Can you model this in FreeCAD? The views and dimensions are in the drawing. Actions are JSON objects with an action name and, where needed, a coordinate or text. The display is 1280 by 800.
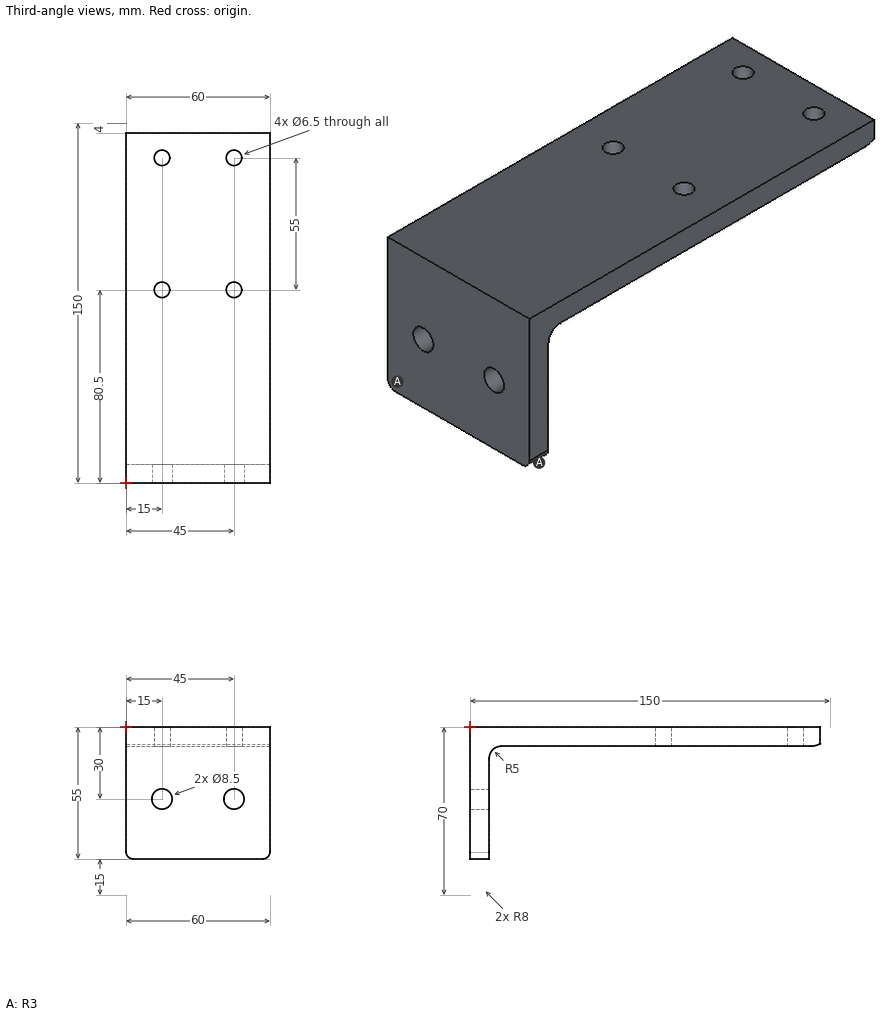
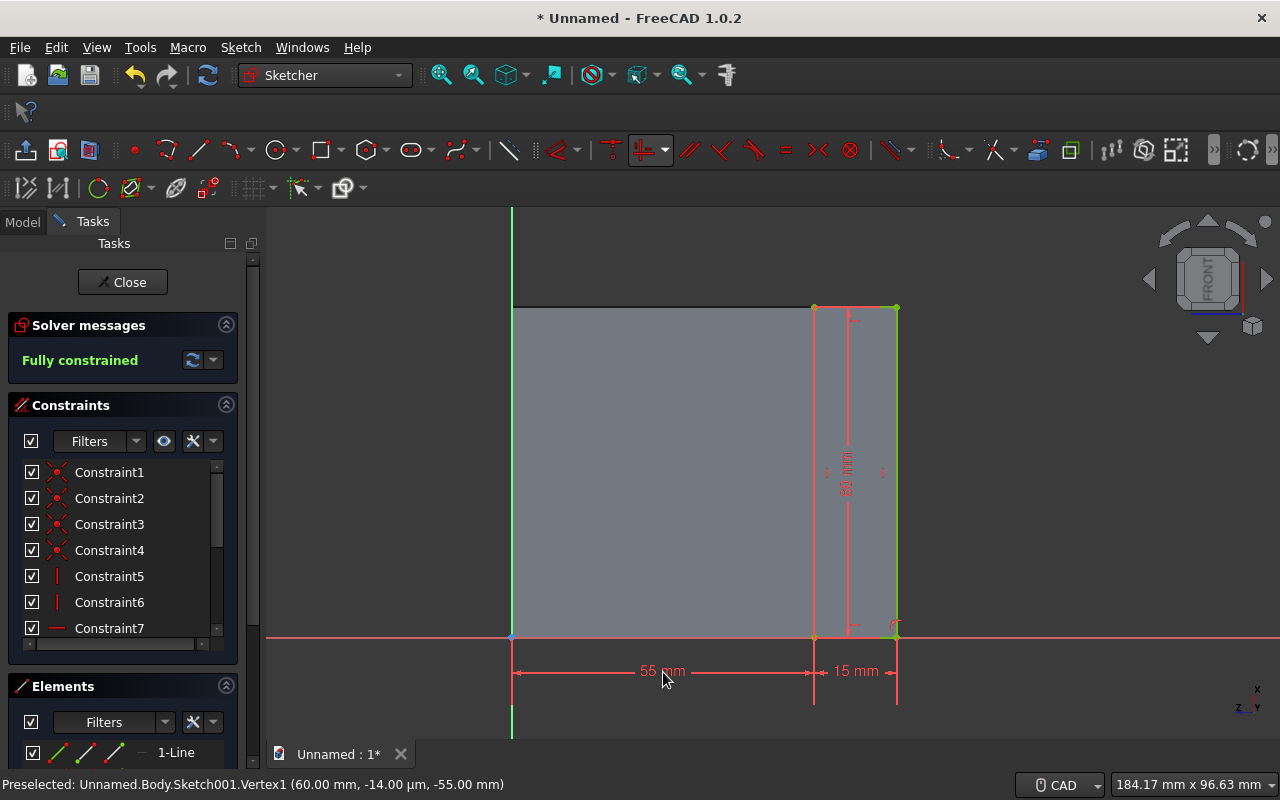
{"action": "left_click", "coordinate": [123, 282]}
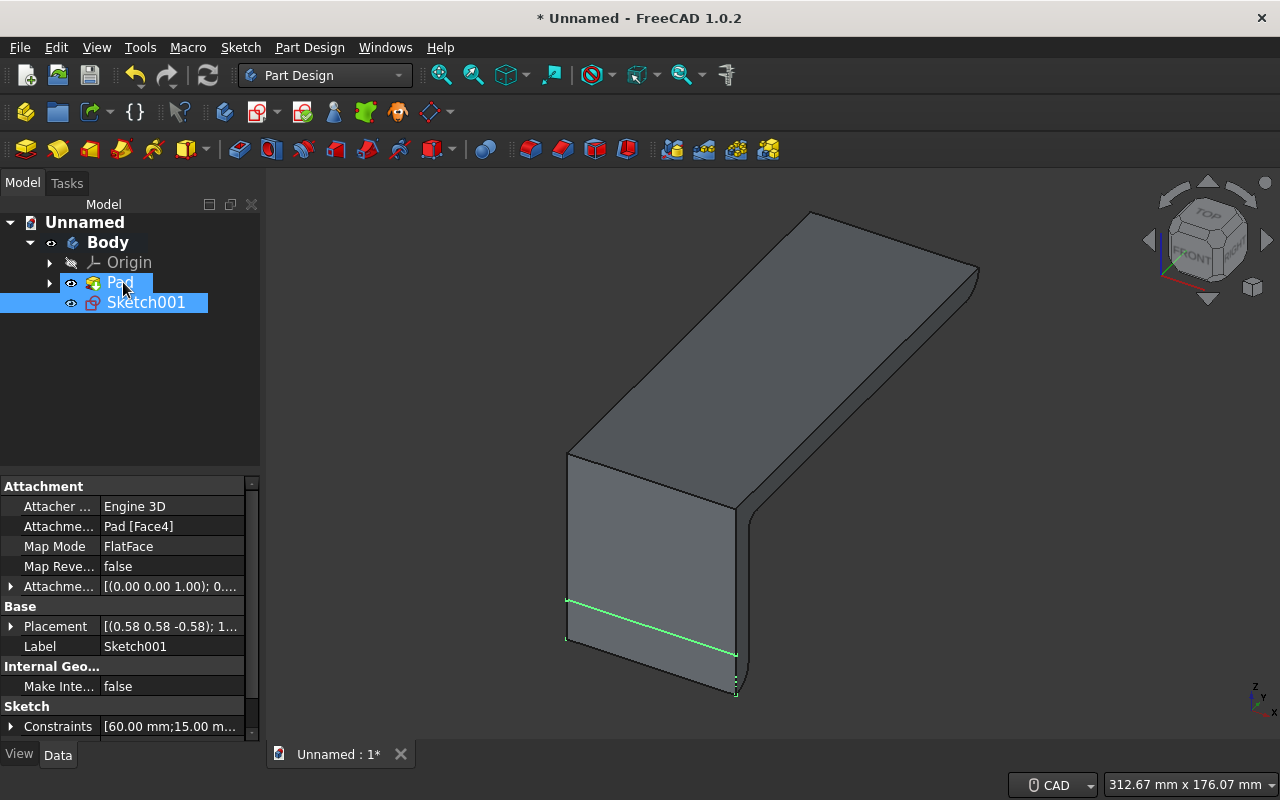
{"action": "left_click", "coordinate": [240, 150]}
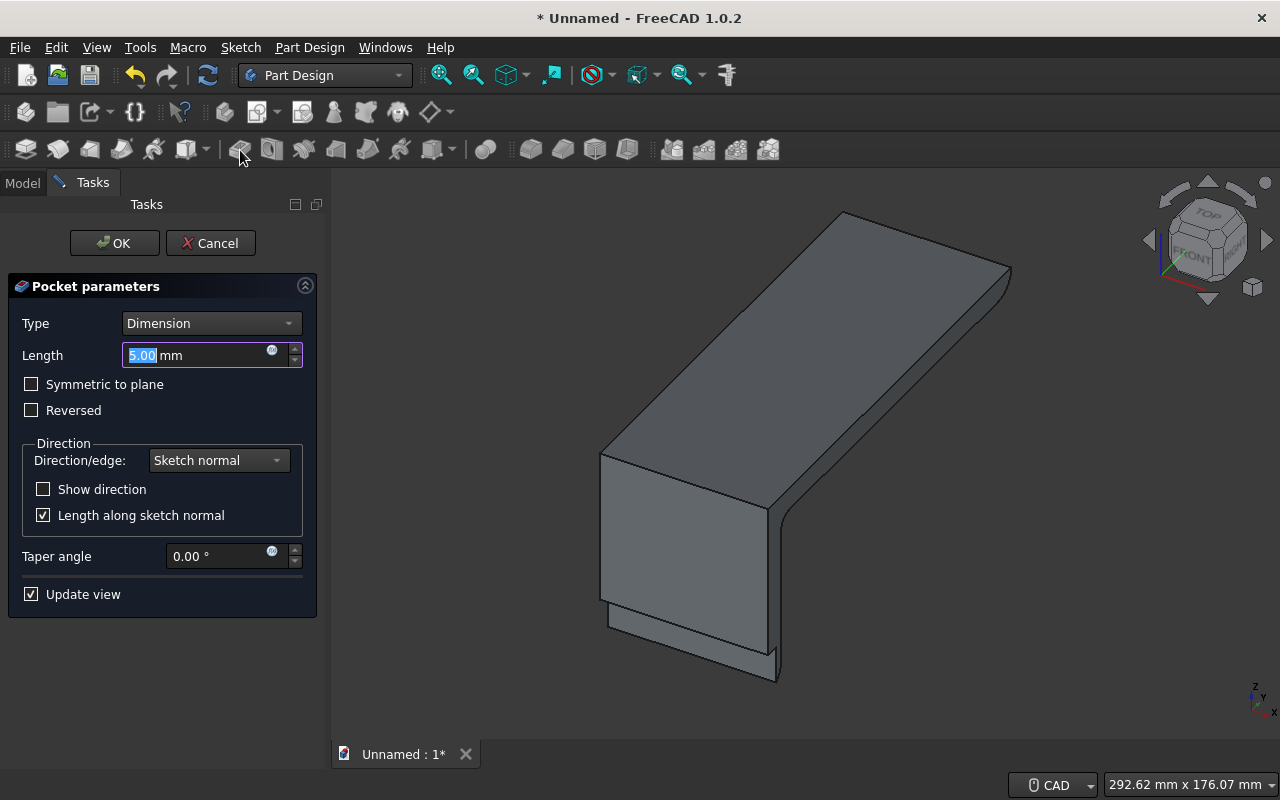
{"action": "left_click", "coordinate": [212, 324]}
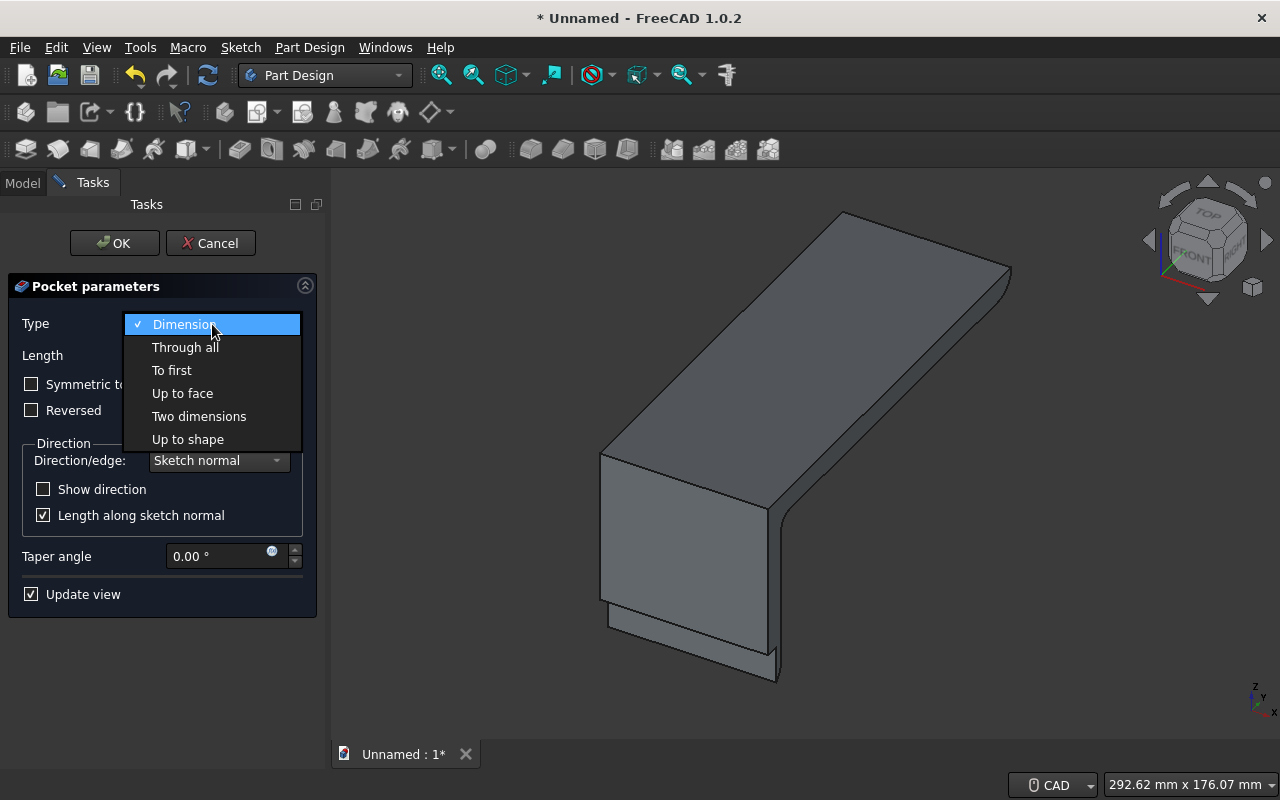
{"action": "left_click", "coordinate": [212, 348]}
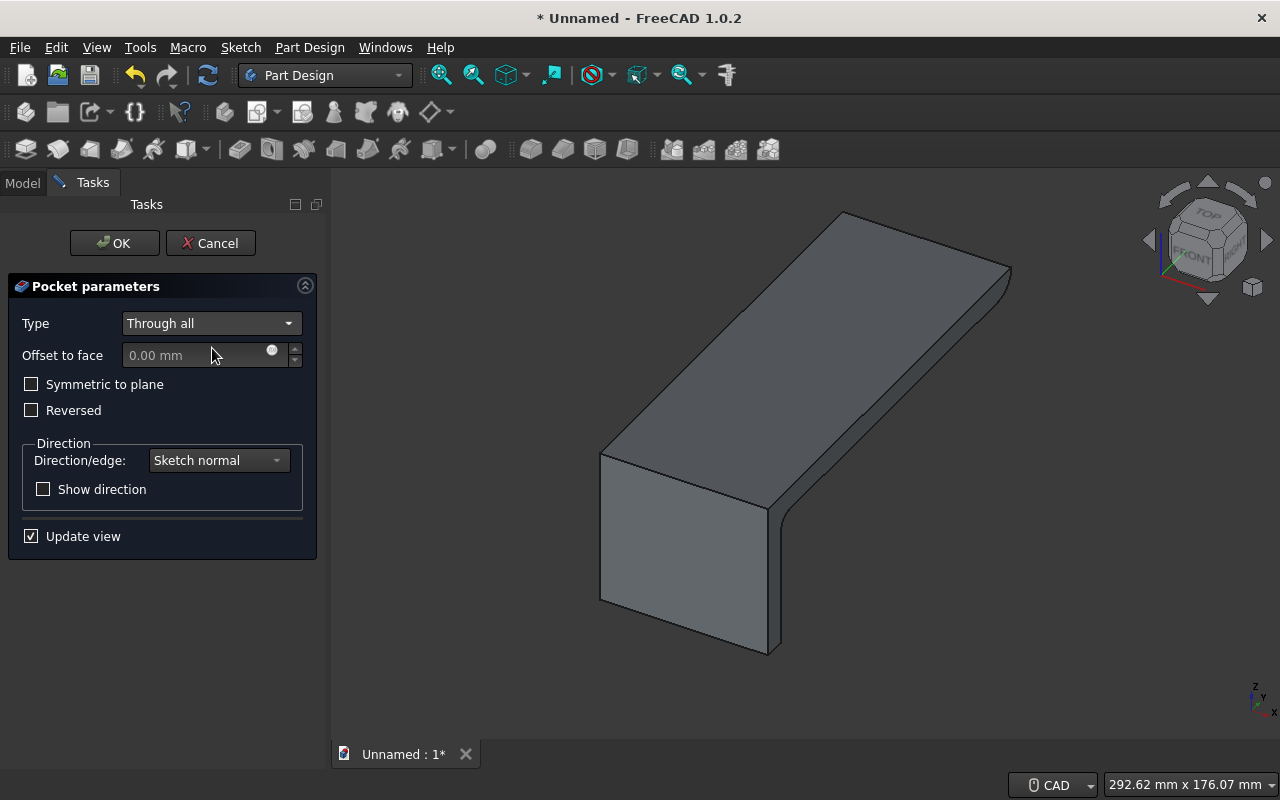
{"action": "left_click", "coordinate": [115, 243]}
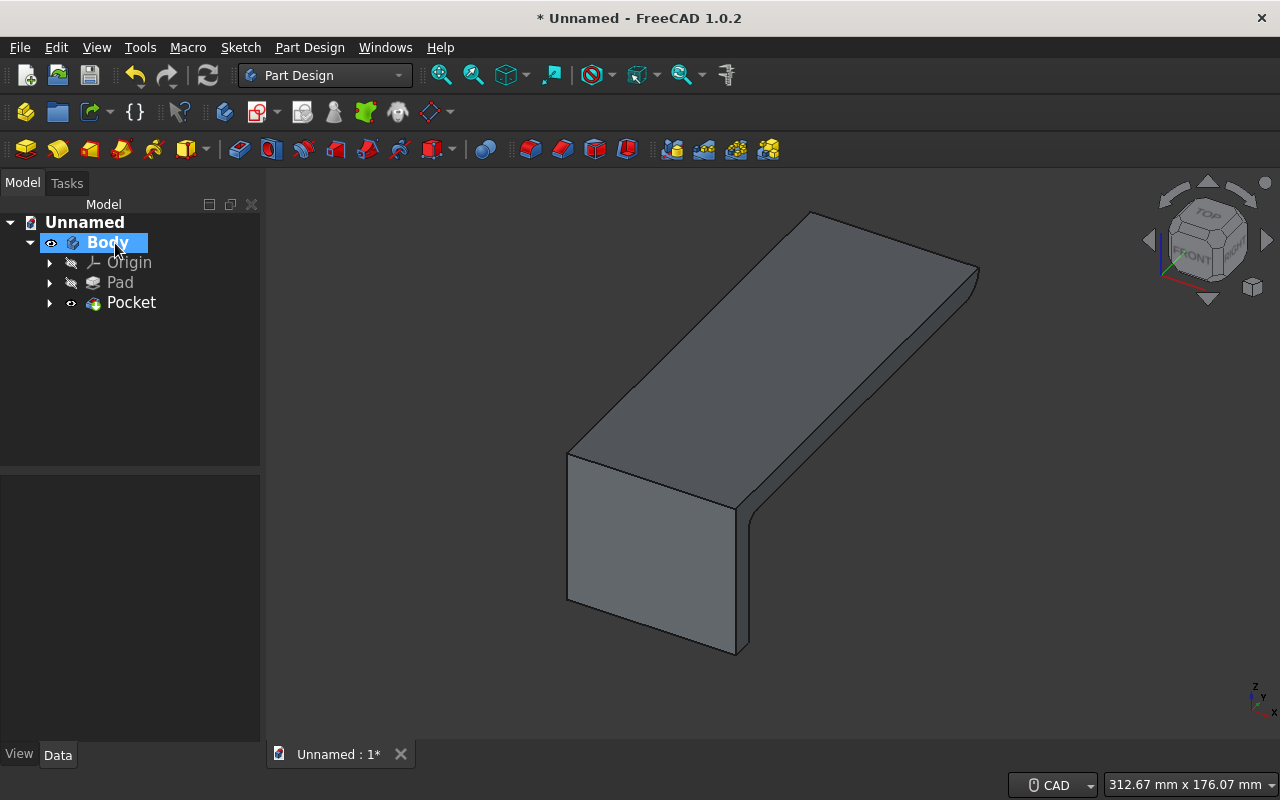
{"action": "left_click", "coordinate": [258, 112]}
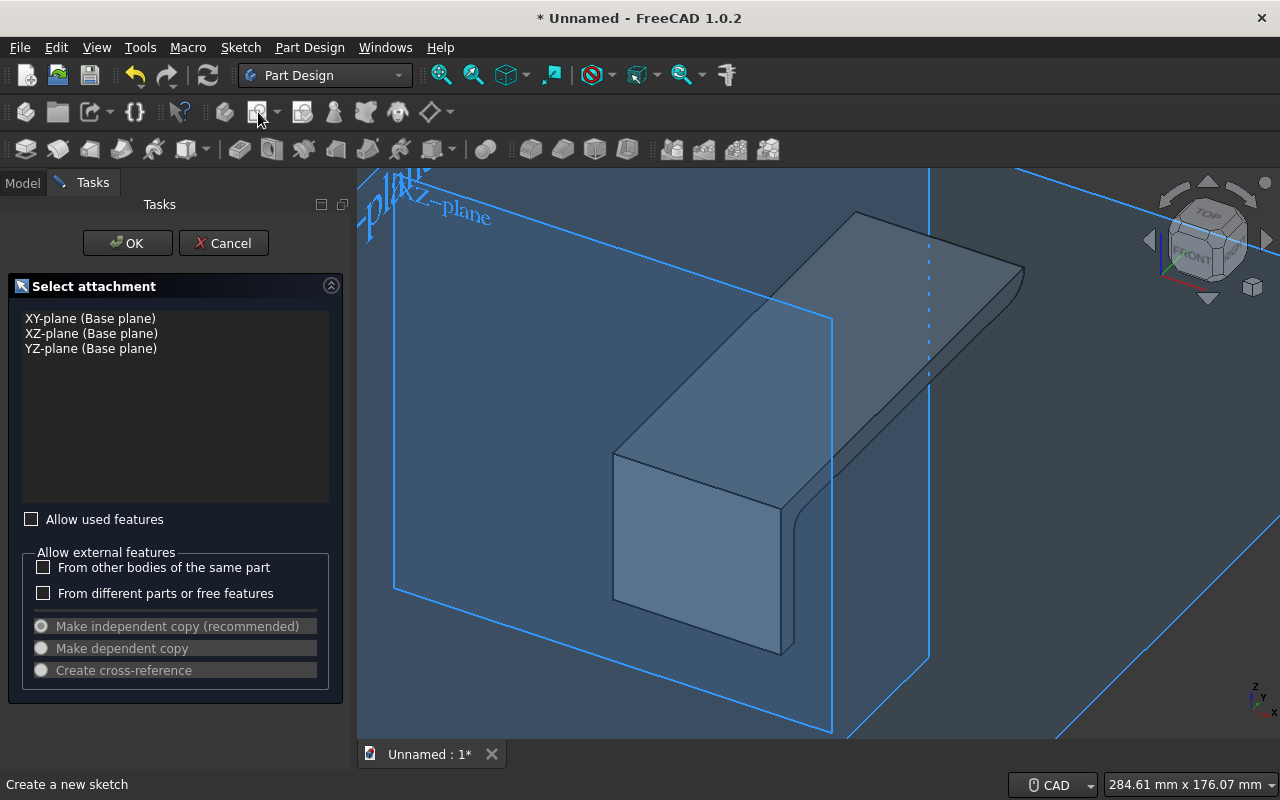
{"action": "left_click", "coordinate": [82, 318]}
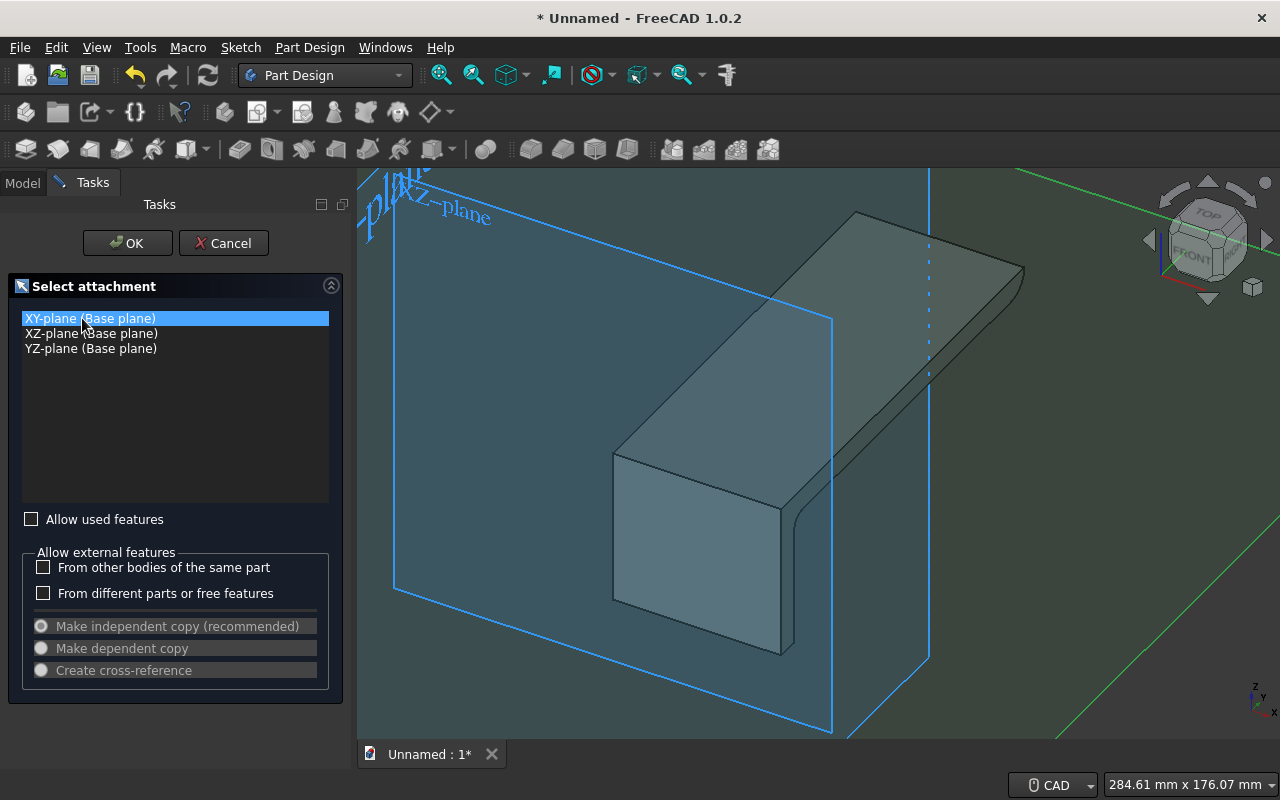
{"action": "left_click", "coordinate": [128, 243]}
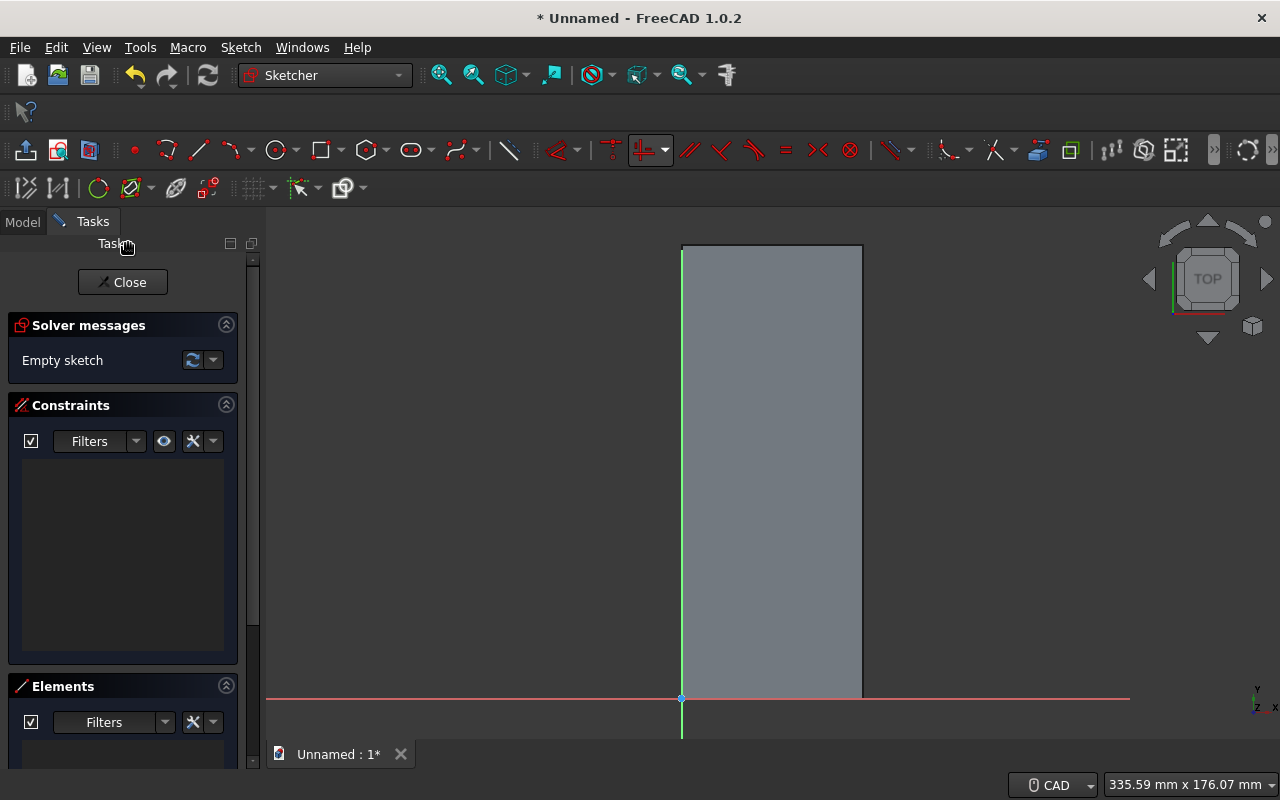
{"action": "scroll", "coordinate": [802, 235], "scroll_direction": "up", "scroll_amount": 6}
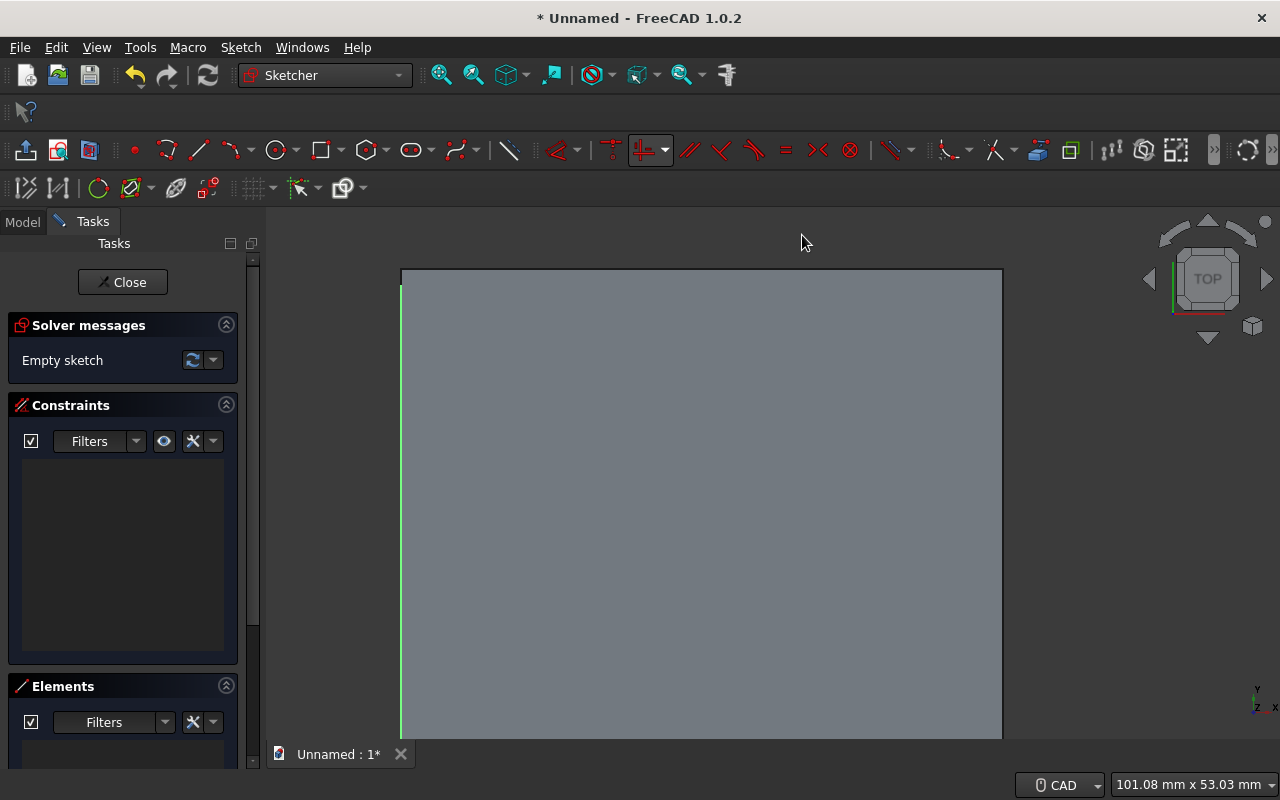
{"action": "key", "text": "g r"}